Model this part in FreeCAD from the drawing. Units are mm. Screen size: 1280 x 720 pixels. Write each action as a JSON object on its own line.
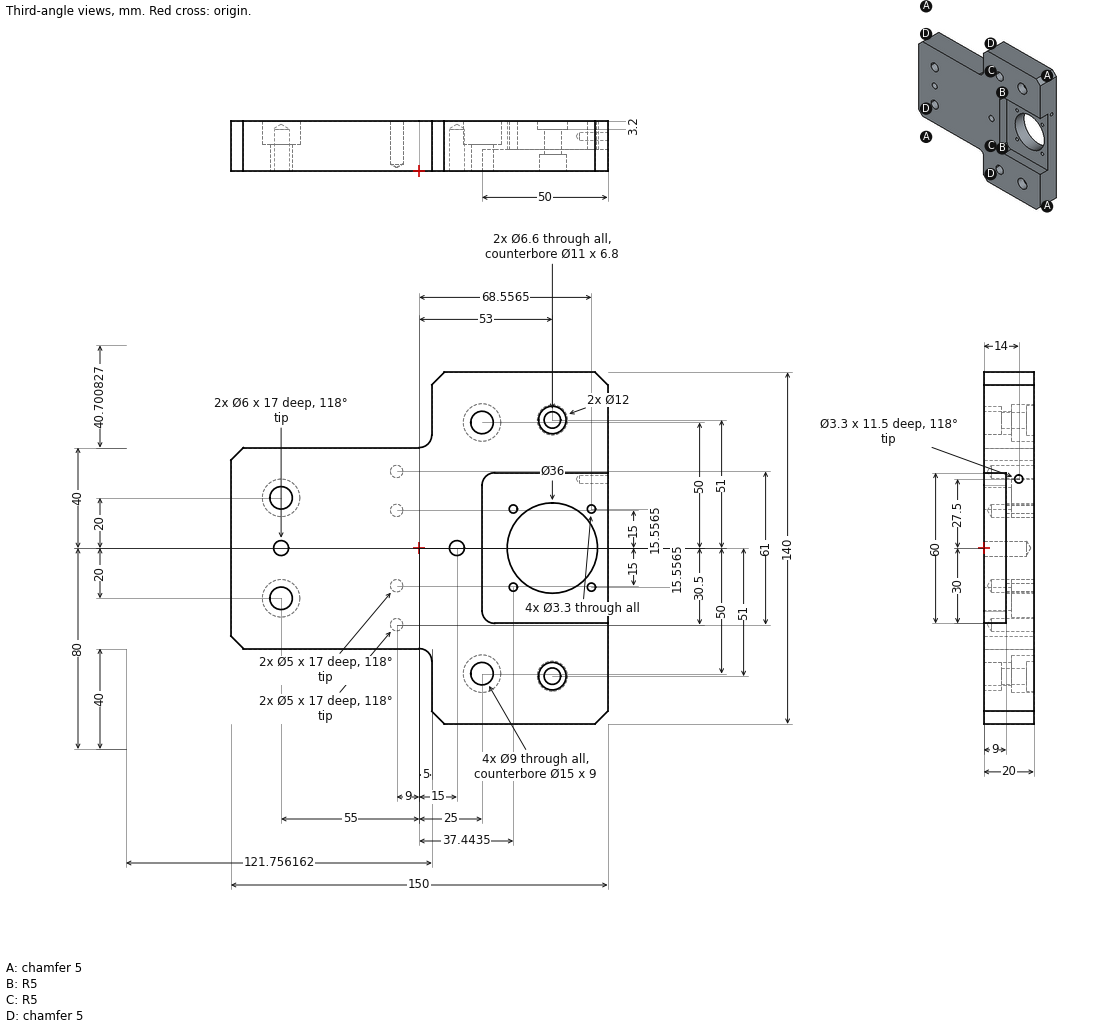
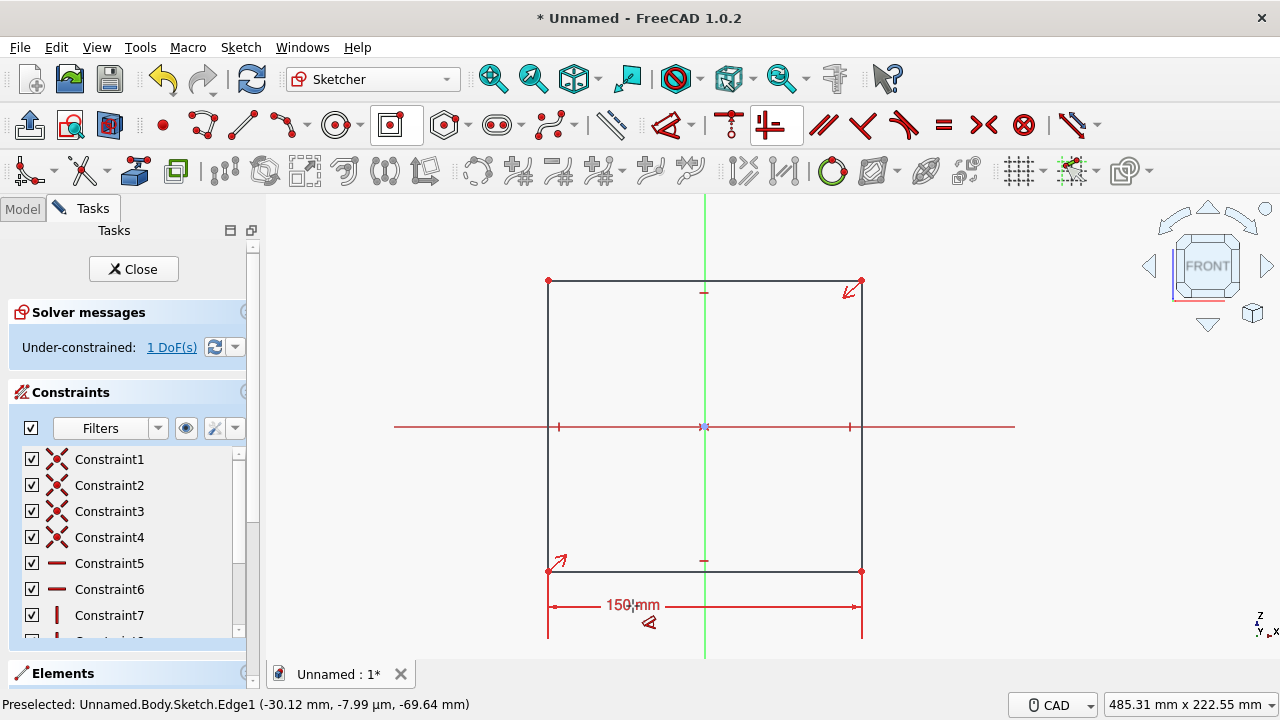
{"action": "left_click", "coordinate": [862, 485]}
{"action": "left_click", "coordinate": [896, 360]}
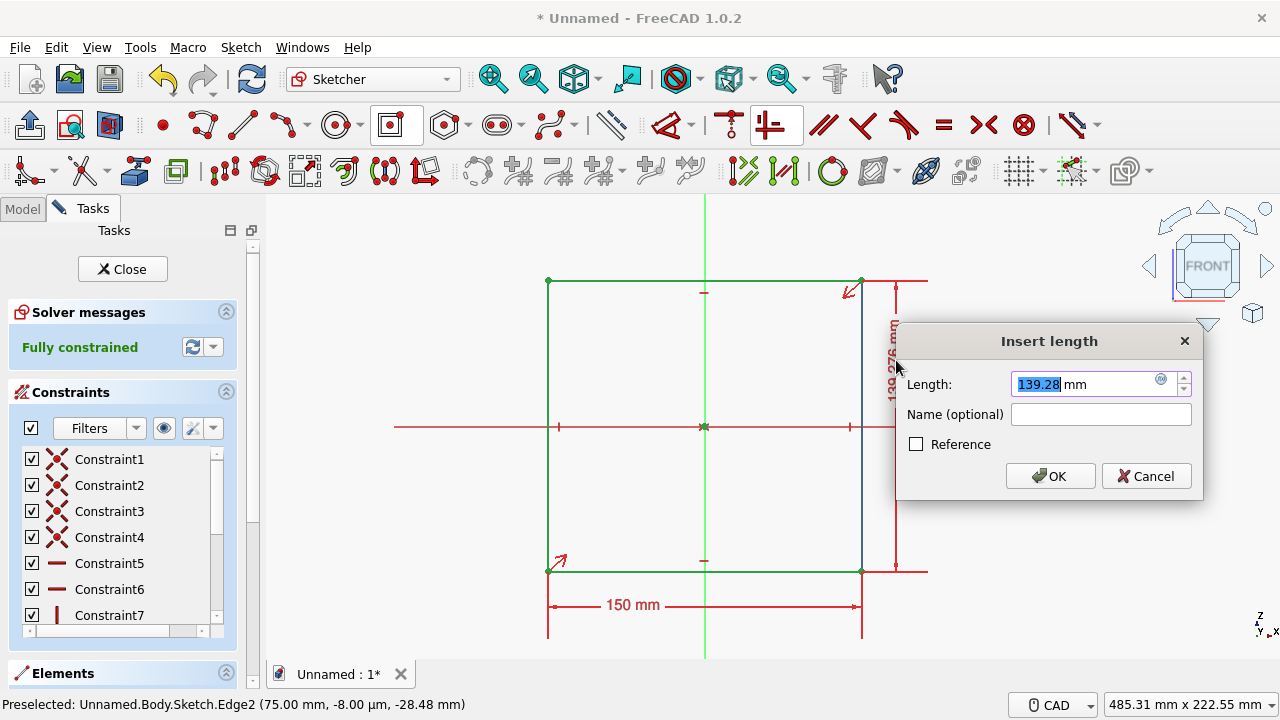
{"action": "type", "text": "140"}
{"action": "key", "text": "Return"}
{"action": "key", "text": "Escape"}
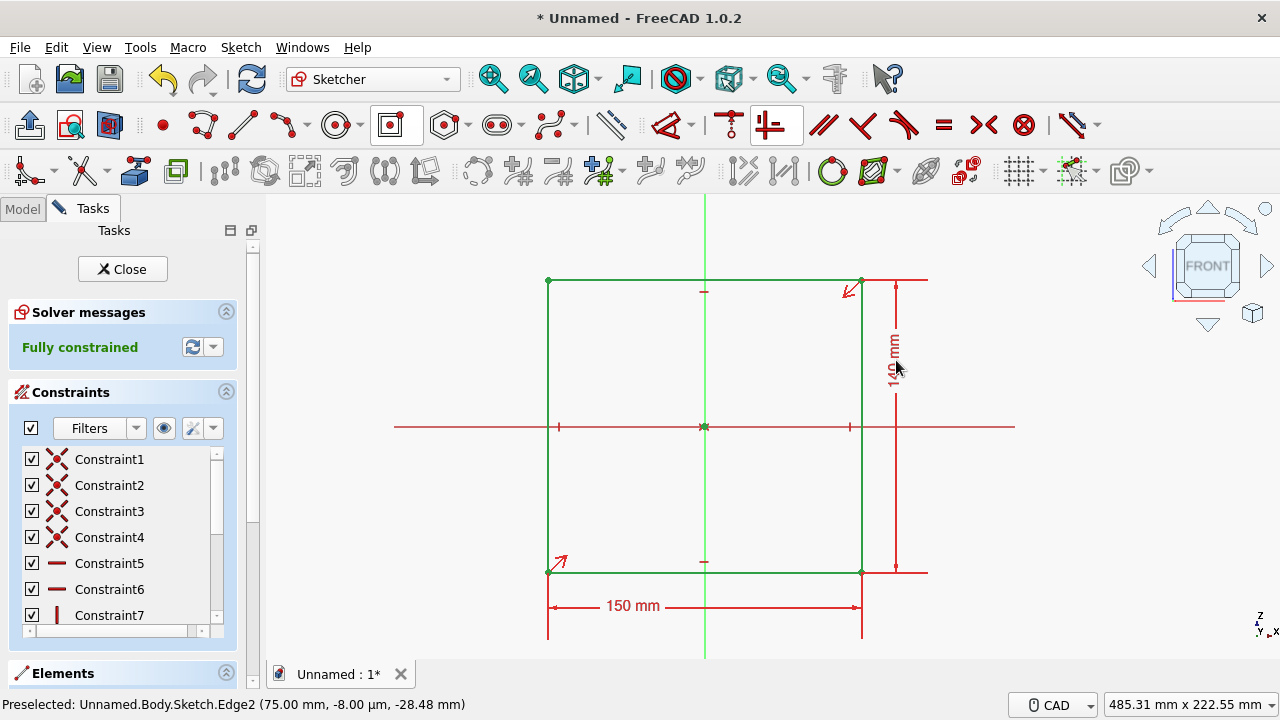
{"action": "left_click", "coordinate": [123, 269]}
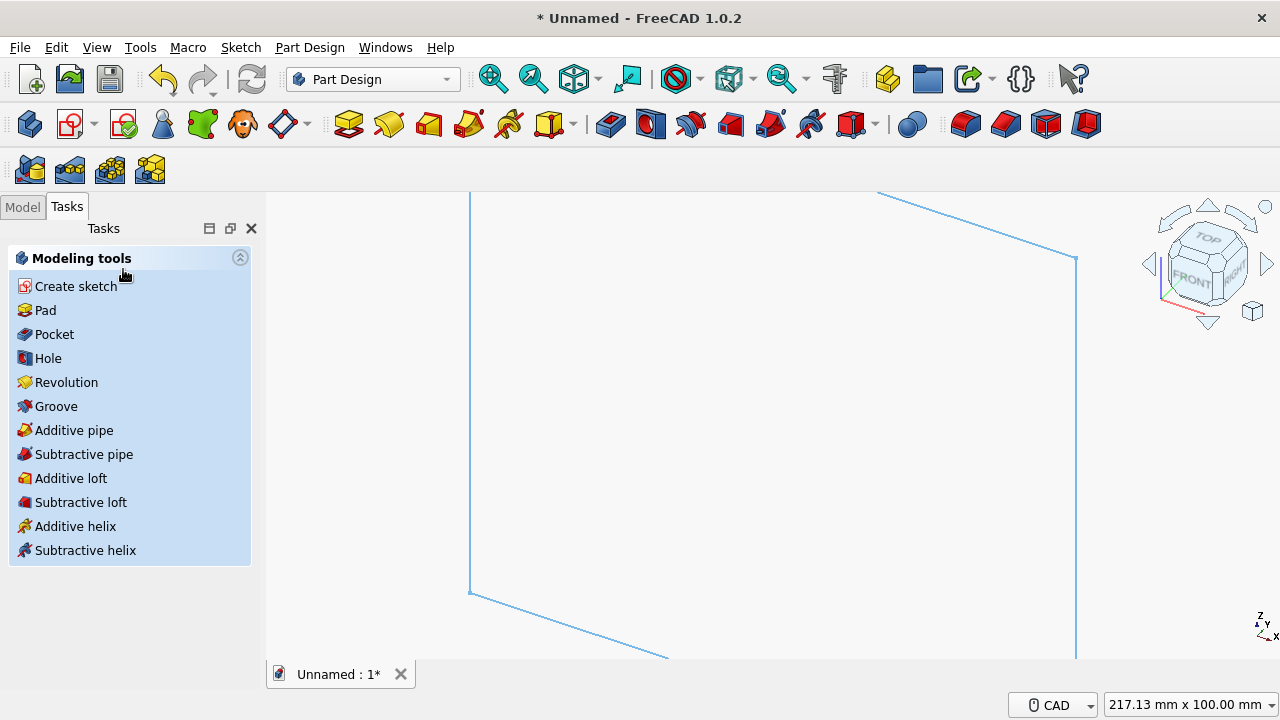
{"action": "left_click", "coordinate": [350, 124]}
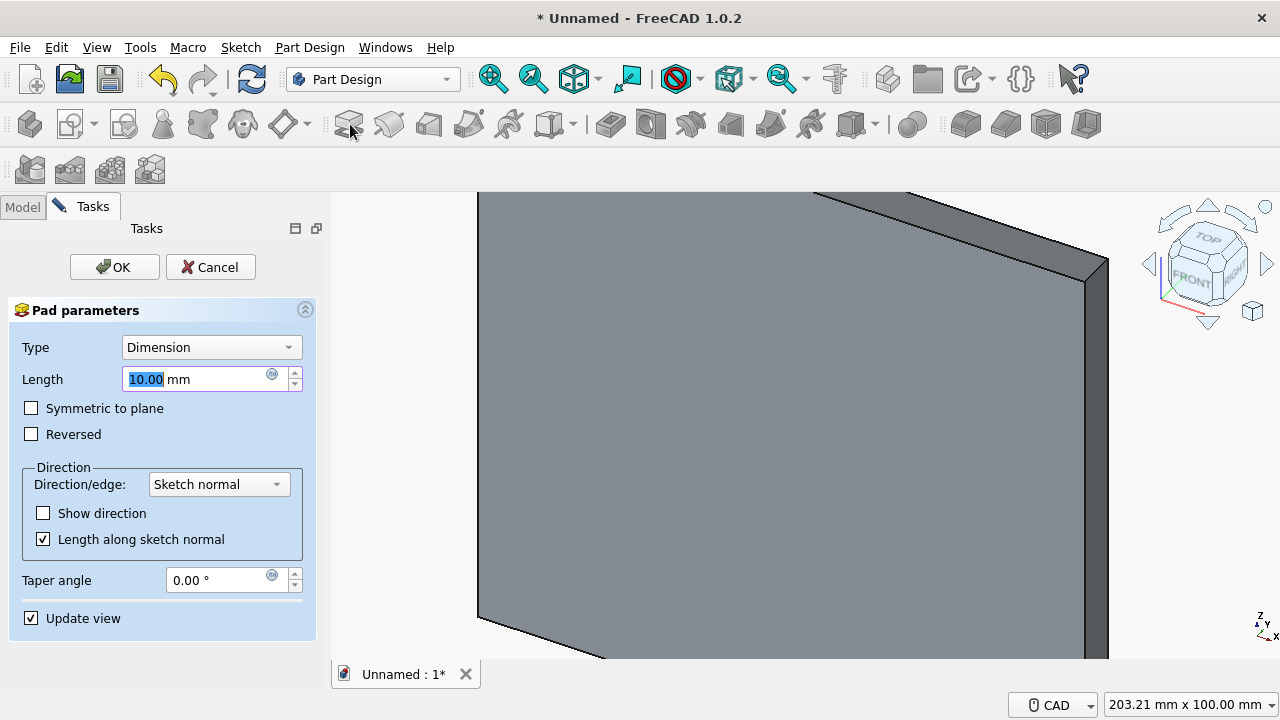
{"action": "type", "text": "20"}
{"action": "key", "text": "Tab"}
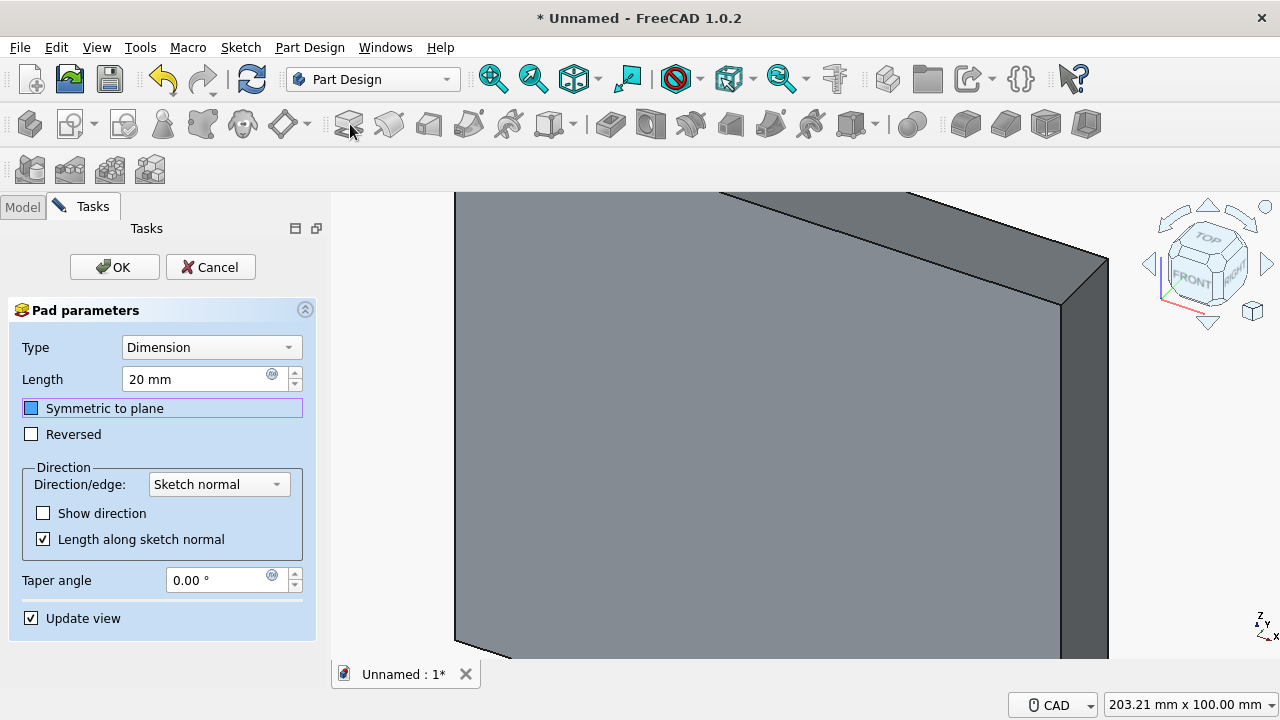
{"action": "left_click", "coordinate": [30, 434]}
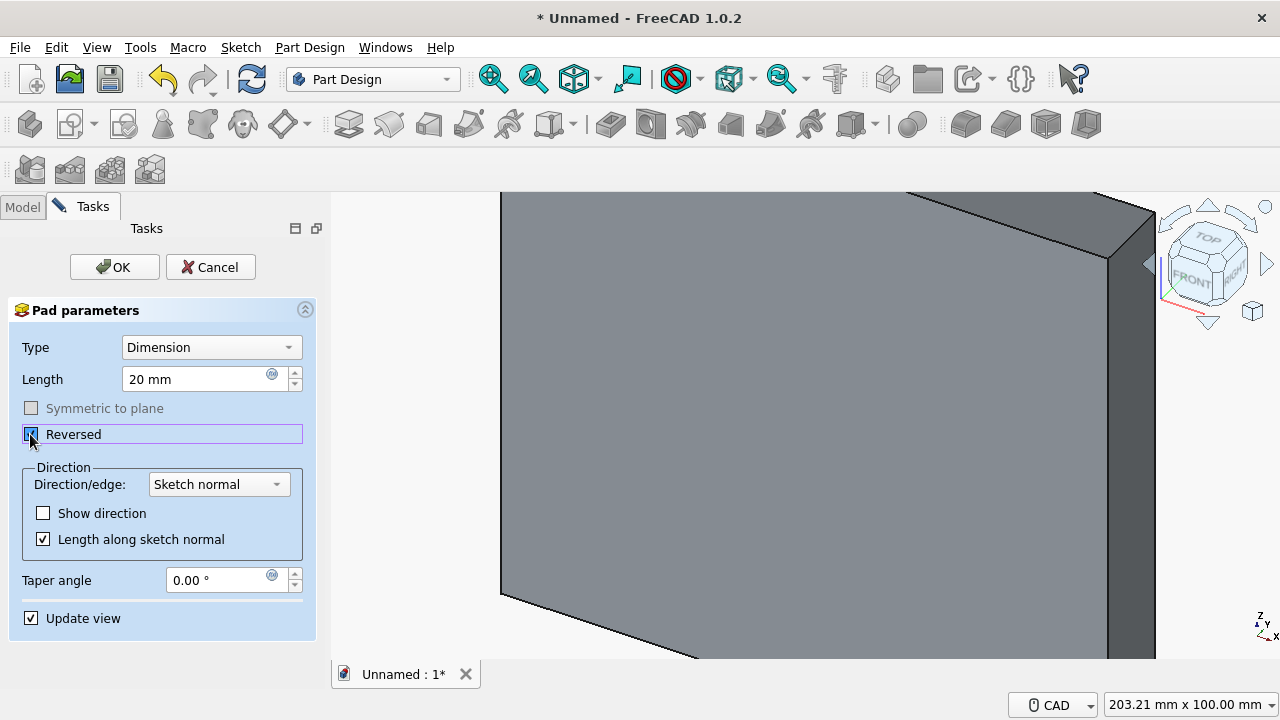
{"action": "left_click", "coordinate": [115, 267]}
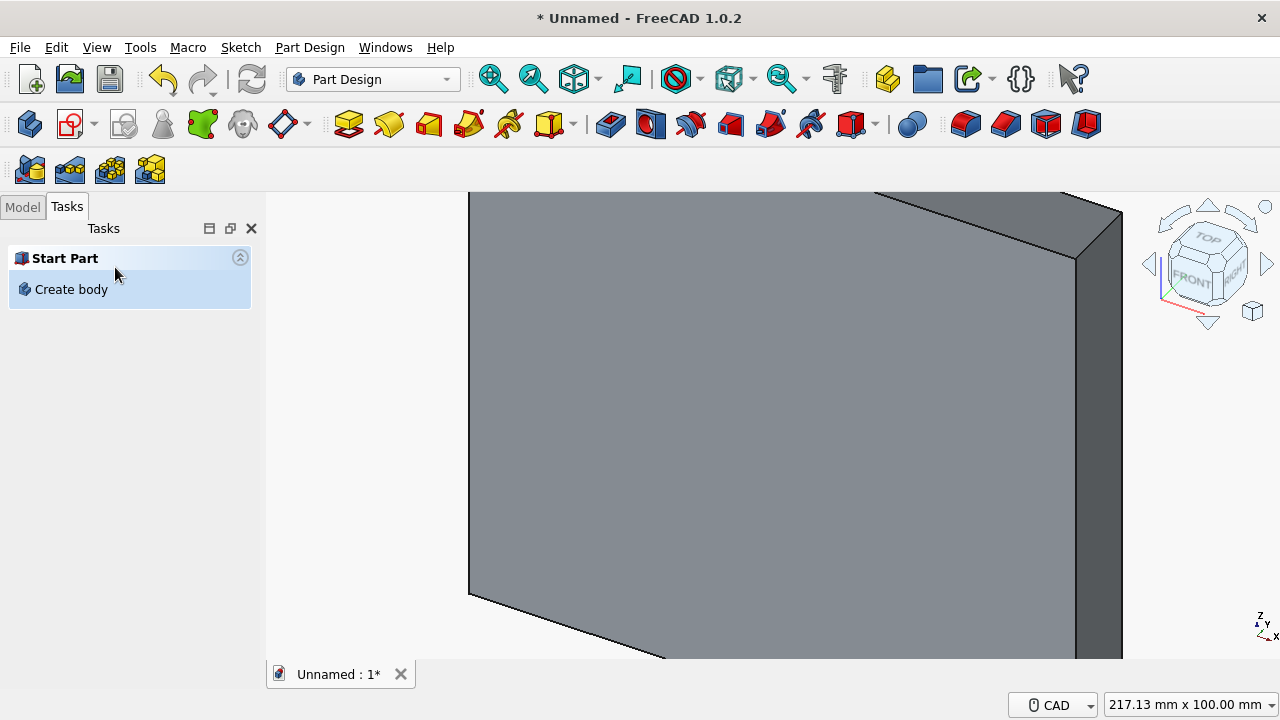
{"action": "left_click", "coordinate": [494, 80]}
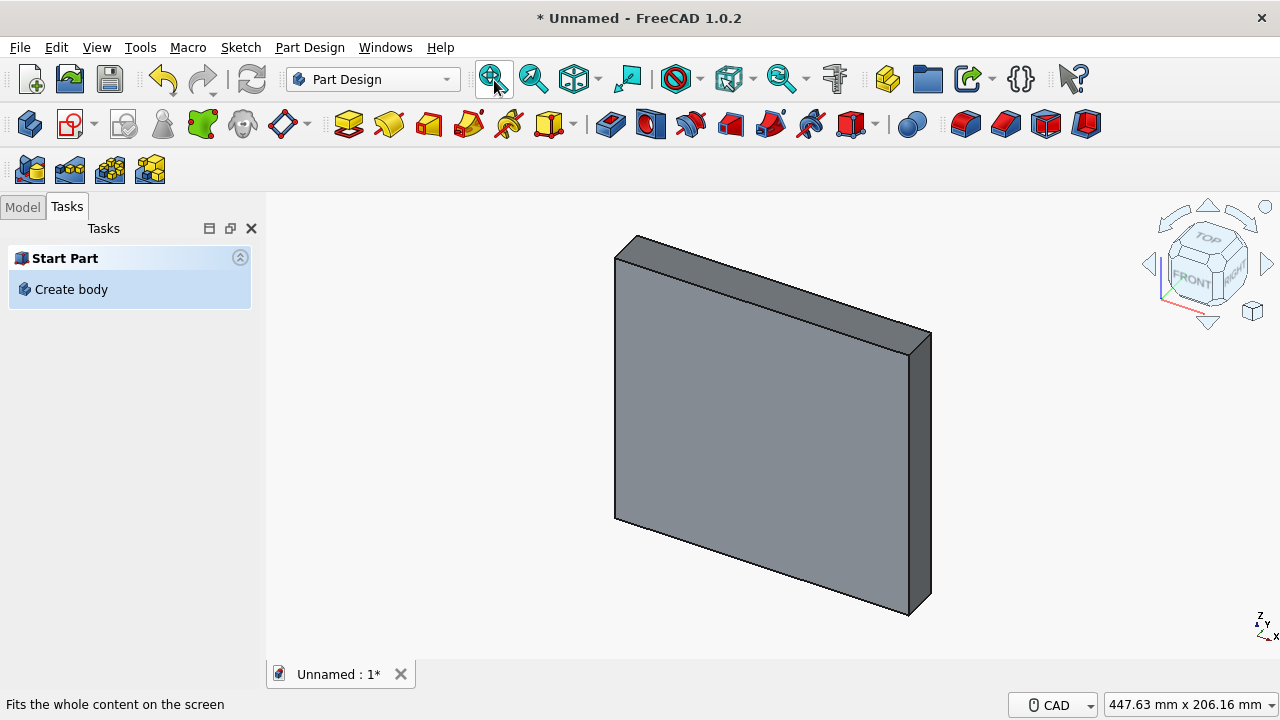
{"action": "left_click", "coordinate": [920, 343]}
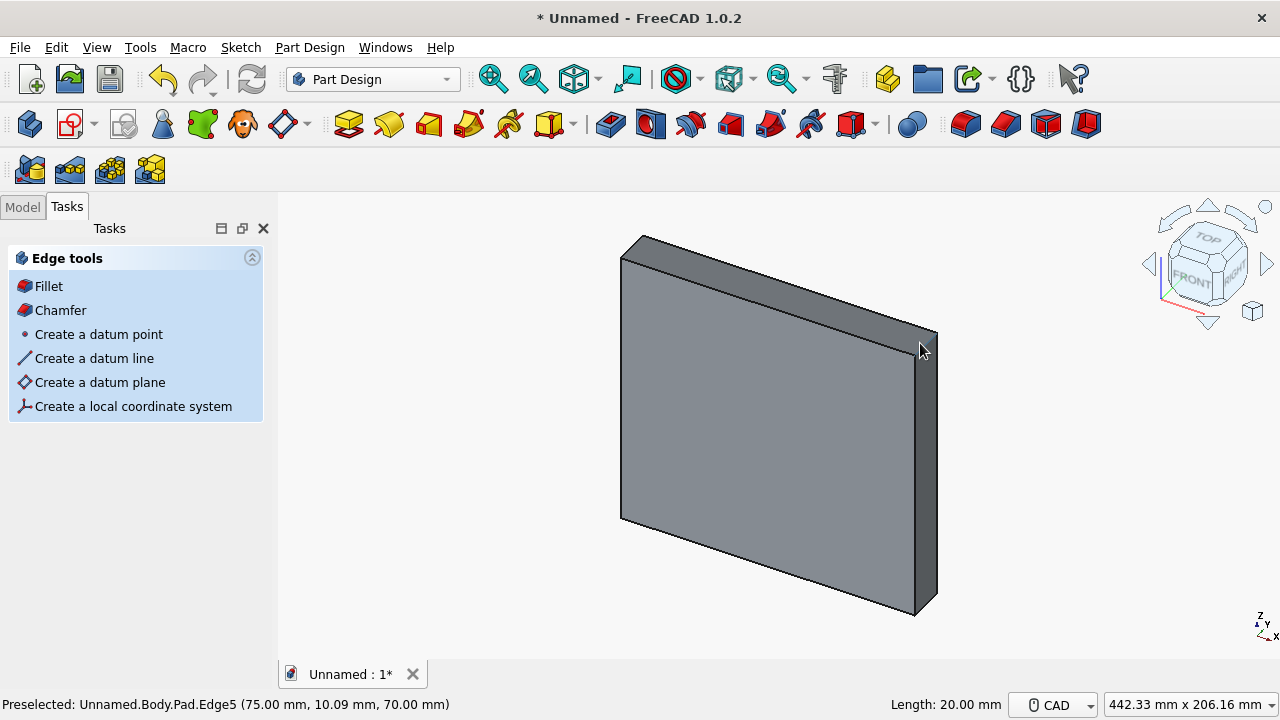
{"action": "key", "text": "0"}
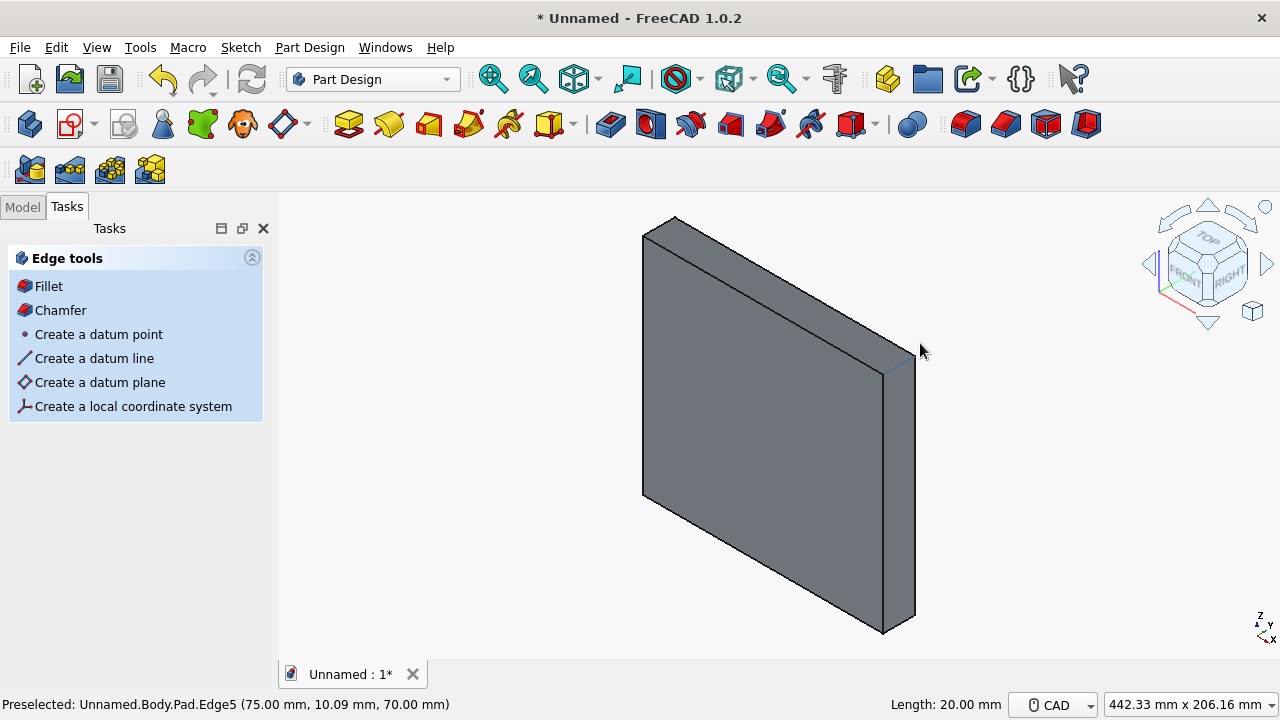
{"action": "key", "text": "2"}